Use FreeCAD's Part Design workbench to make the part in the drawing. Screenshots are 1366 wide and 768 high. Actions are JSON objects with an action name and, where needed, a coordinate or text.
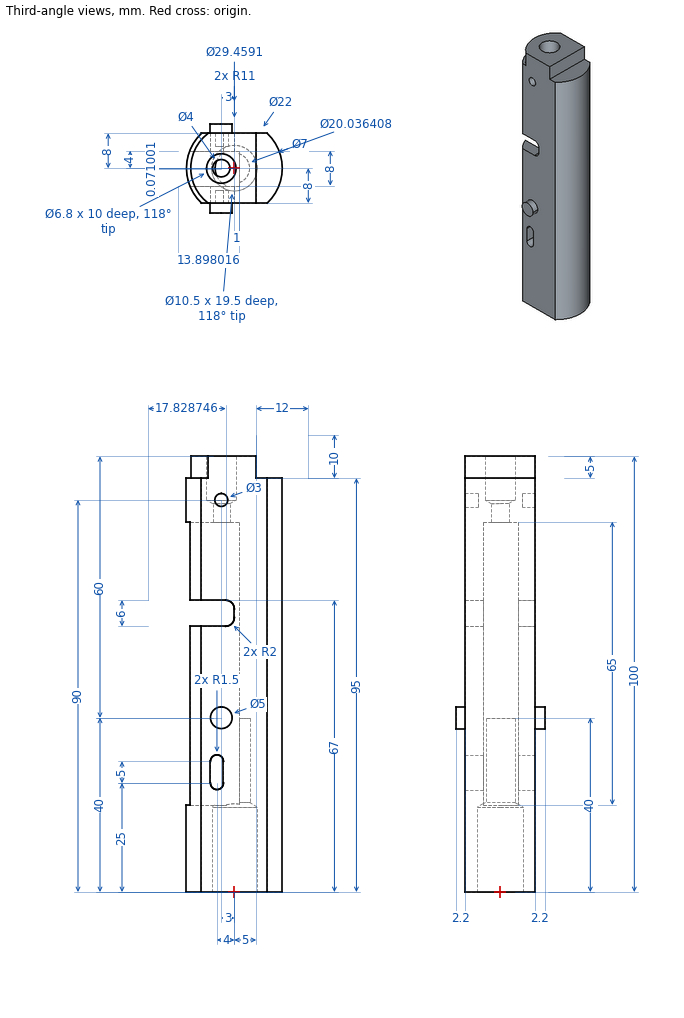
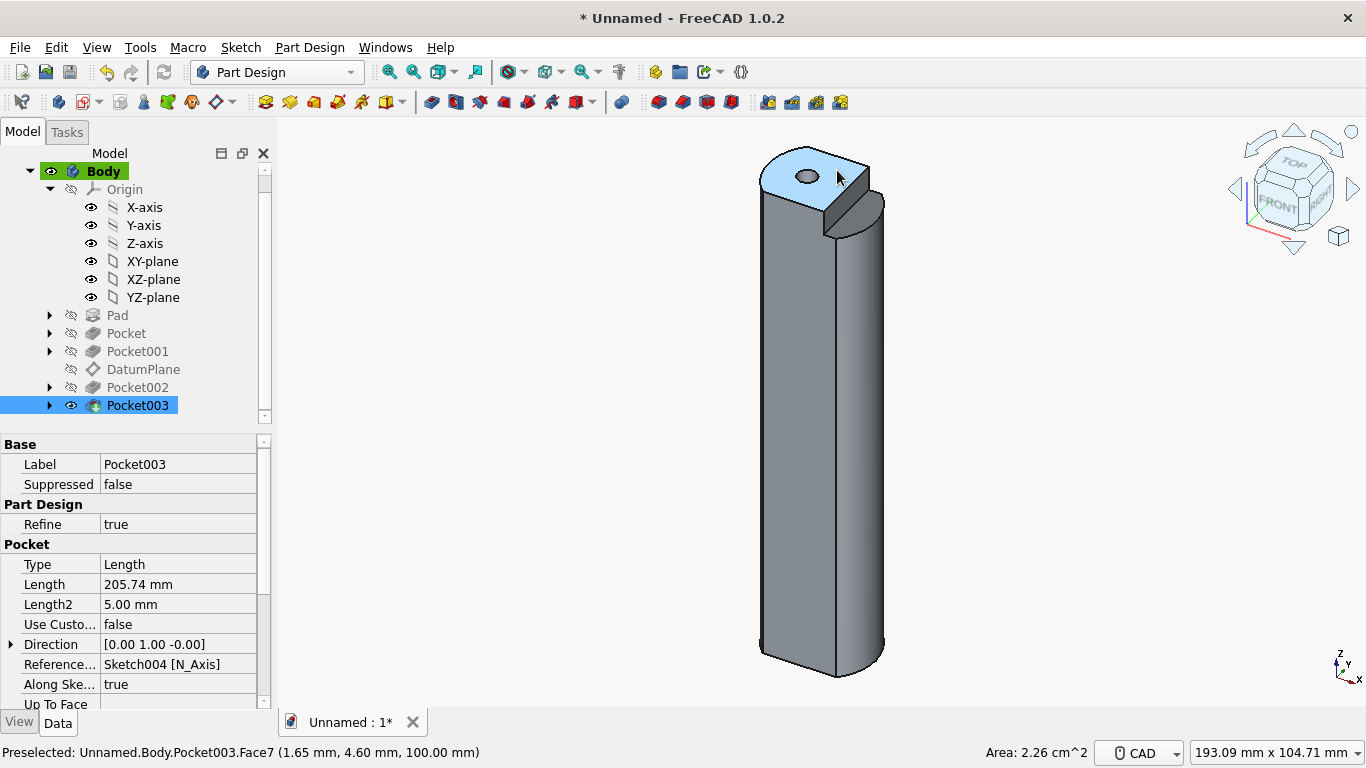
{"action": "left_click", "coordinate": [84, 102]}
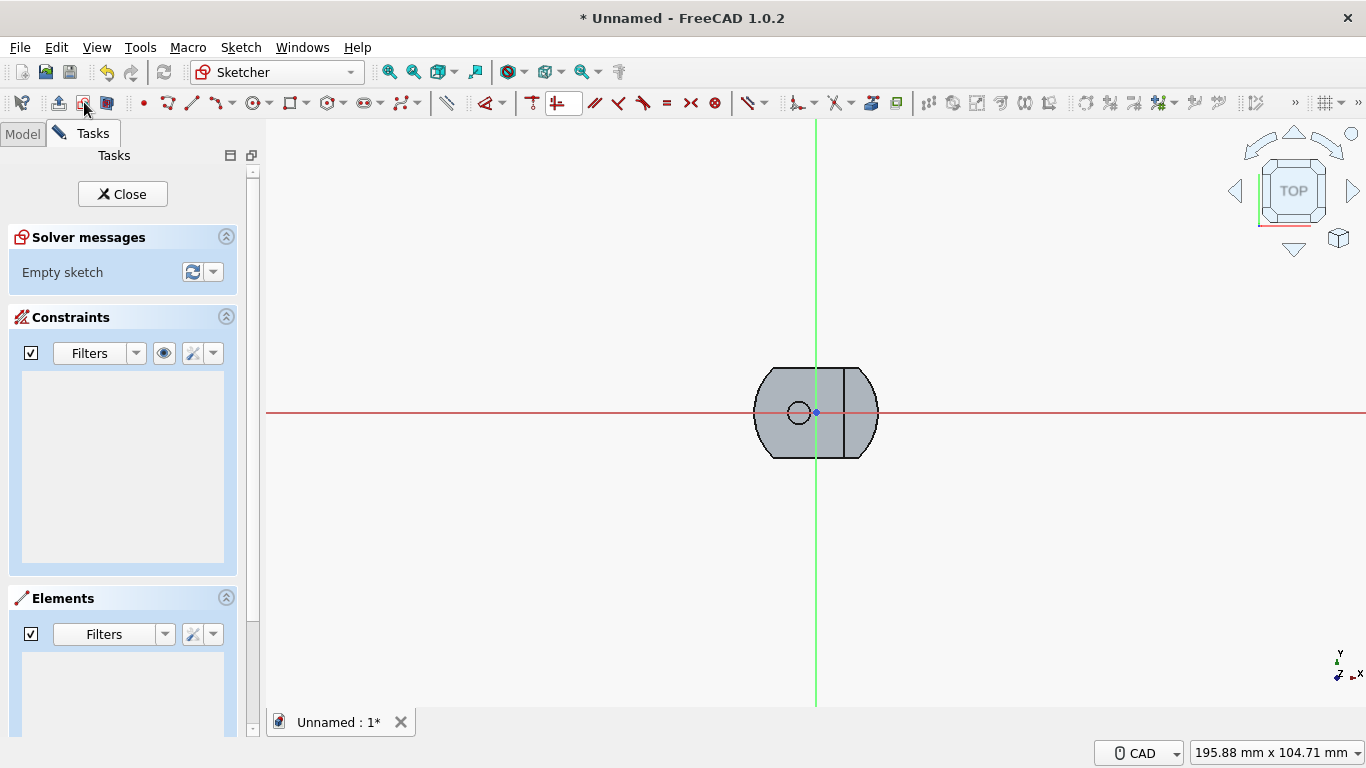
{"action": "scroll", "coordinate": [806, 413], "scroll_direction": "up", "scroll_amount": 11}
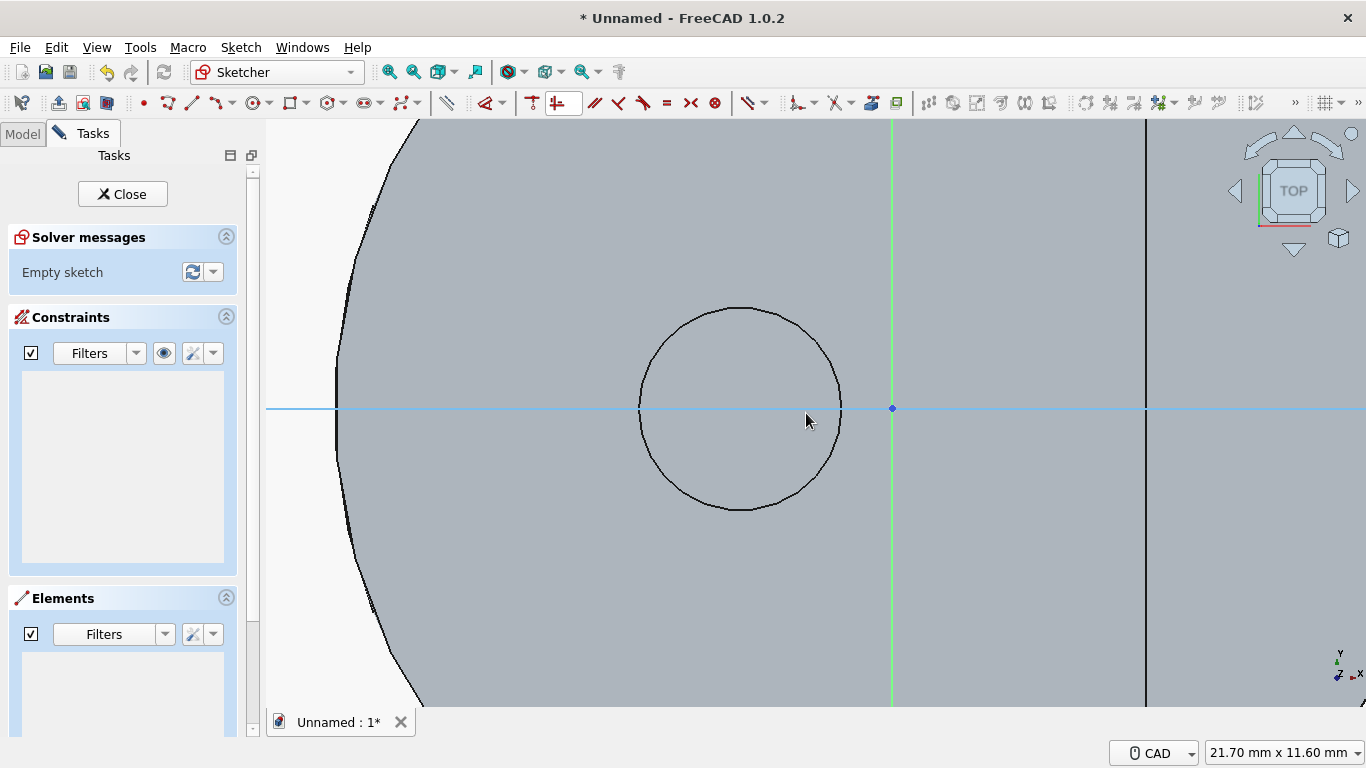
{"action": "left_click", "coordinate": [254, 104]}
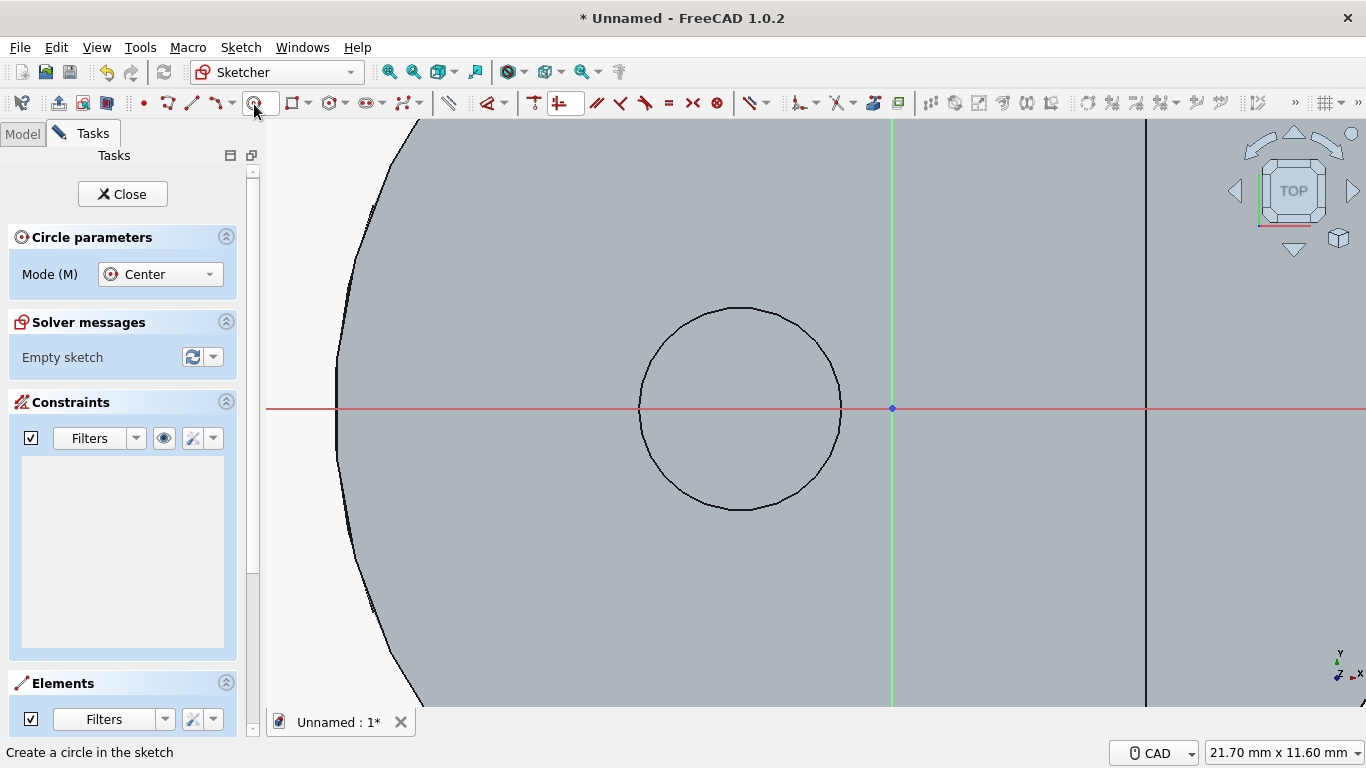
{"action": "scroll", "coordinate": [740, 413], "scroll_direction": "up", "scroll_amount": 8}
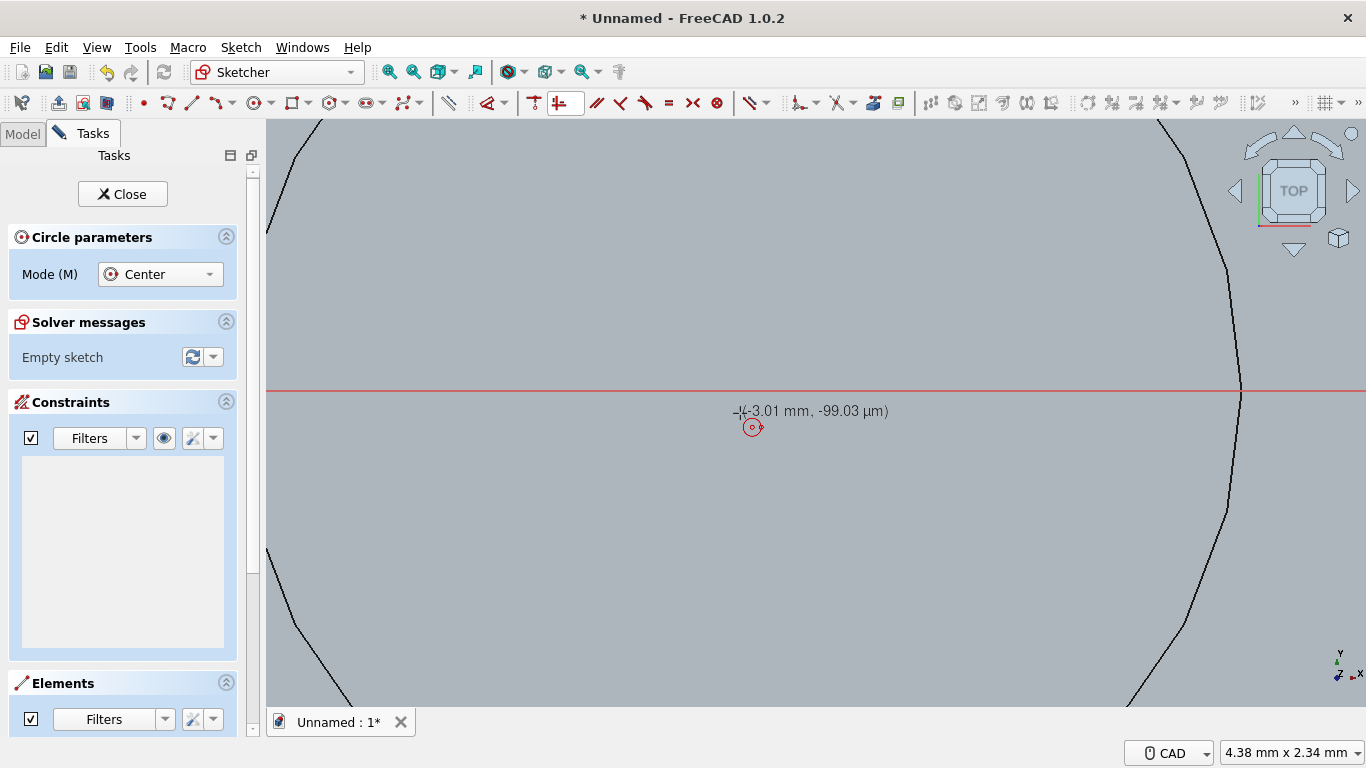
{"action": "left_click", "coordinate": [740, 409]}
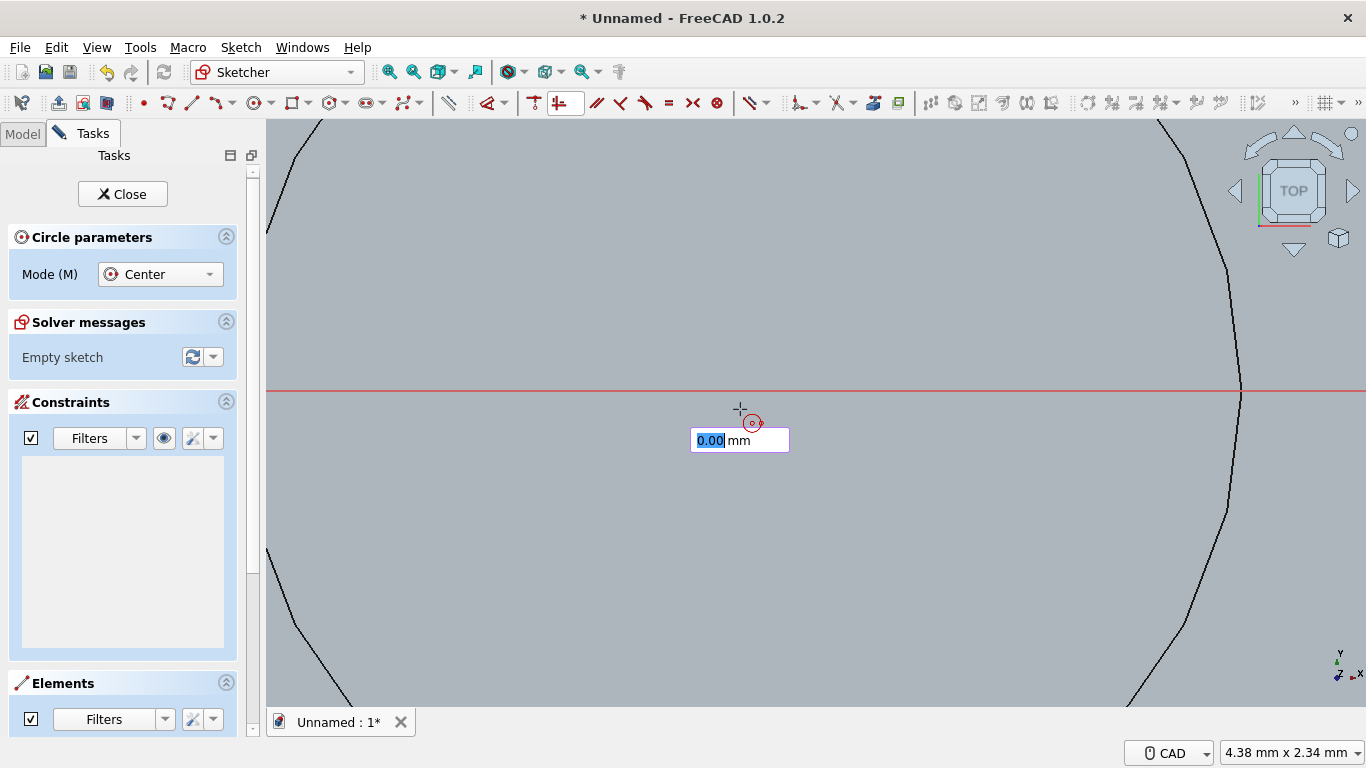
{"action": "scroll", "coordinate": [749, 414], "scroll_direction": "down", "scroll_amount": 8}
{"action": "mouse_move", "coordinate": [869, 292]}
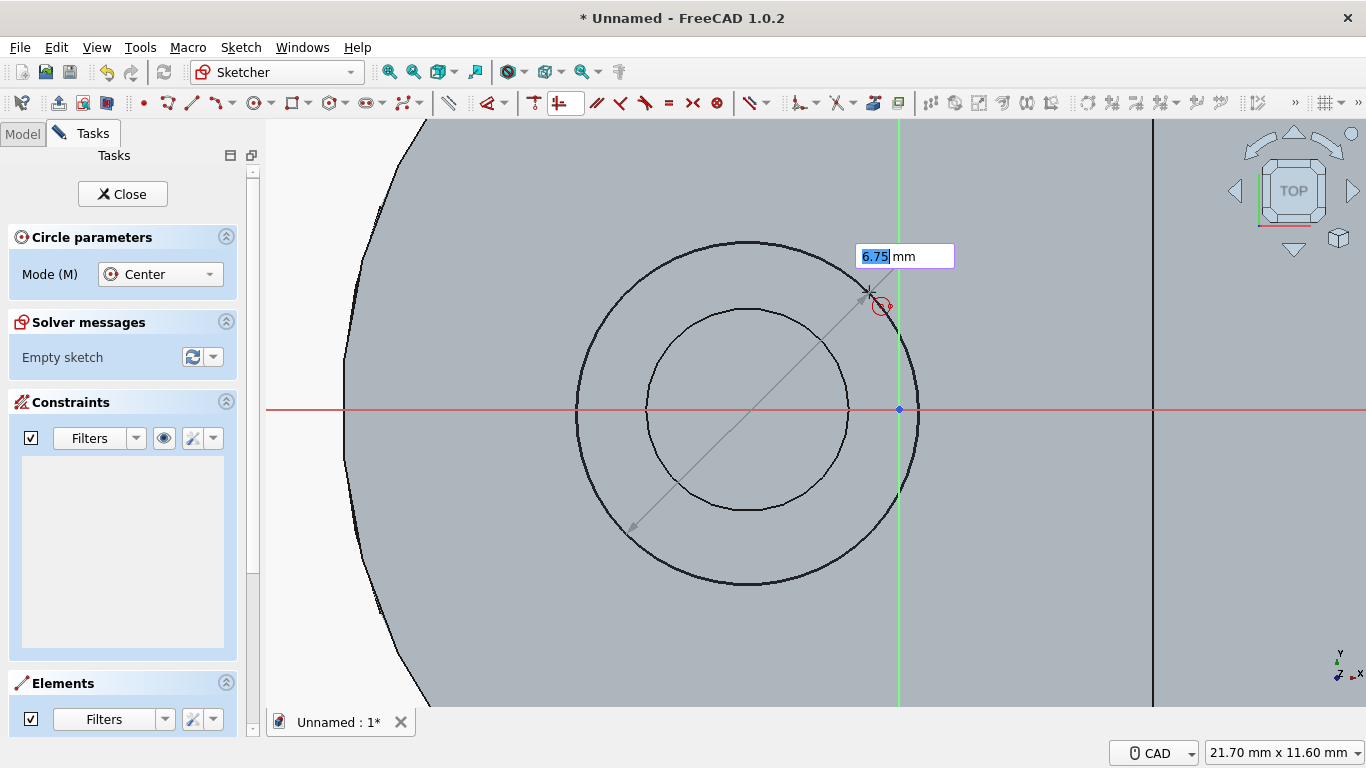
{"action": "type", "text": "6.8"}
{"action": "key", "text": "Return"}
{"action": "key", "text": "Escape"}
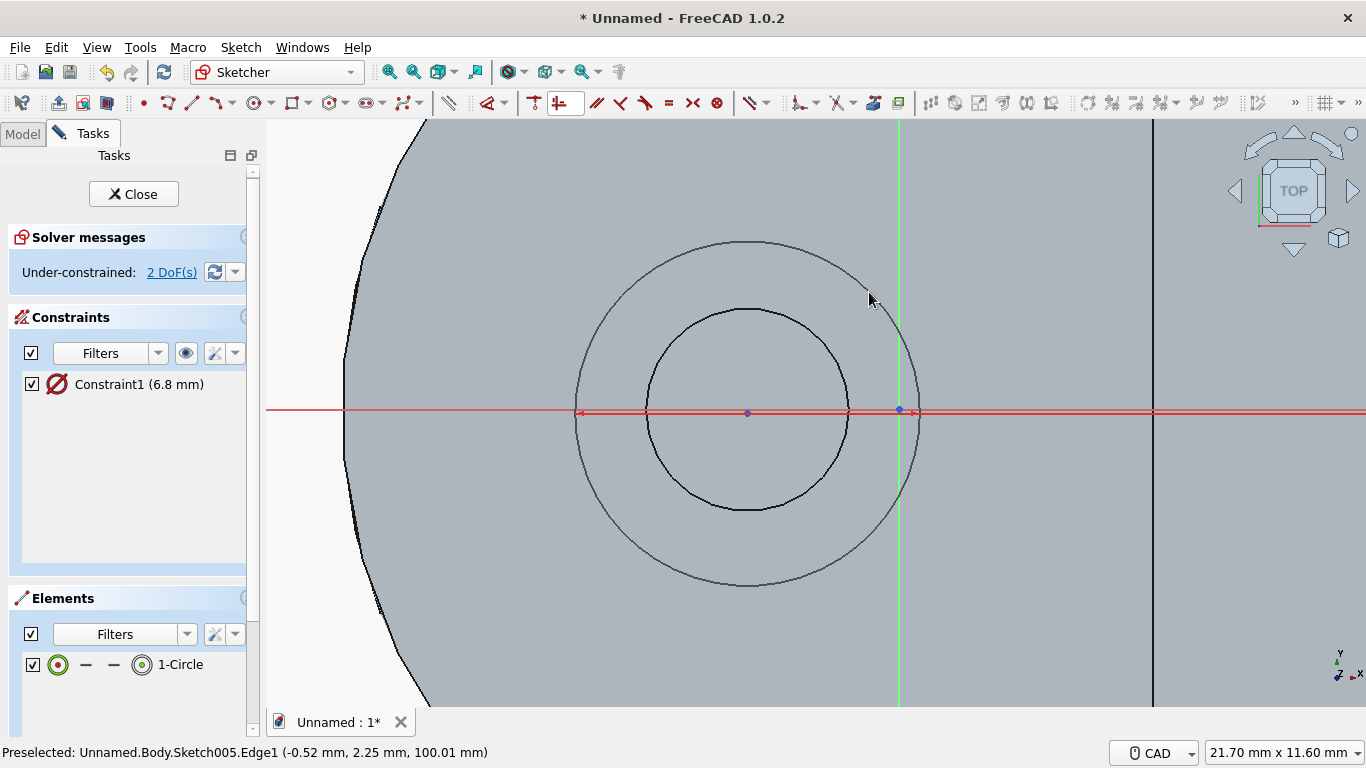
{"action": "key", "text": "d"}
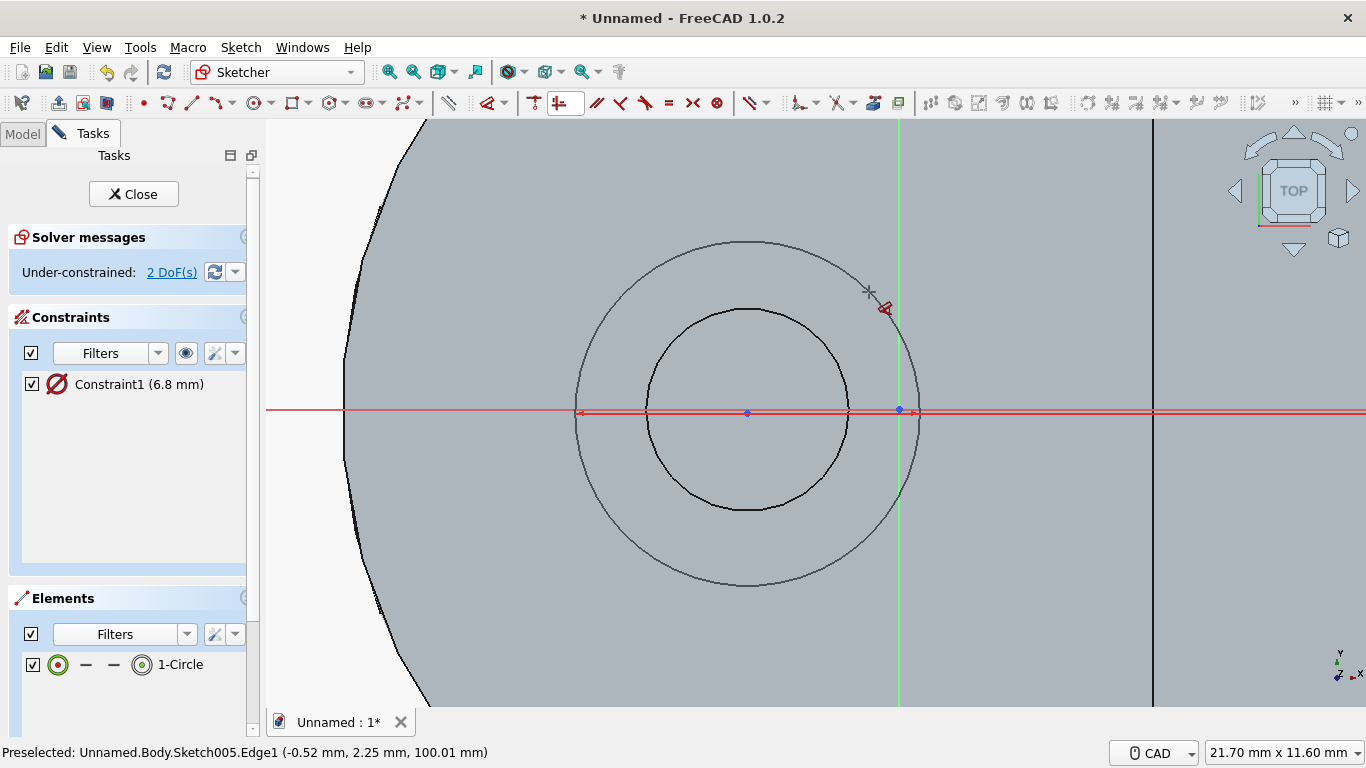
{"action": "left_click", "coordinate": [748, 414]}
{"action": "left_click", "coordinate": [824, 376]}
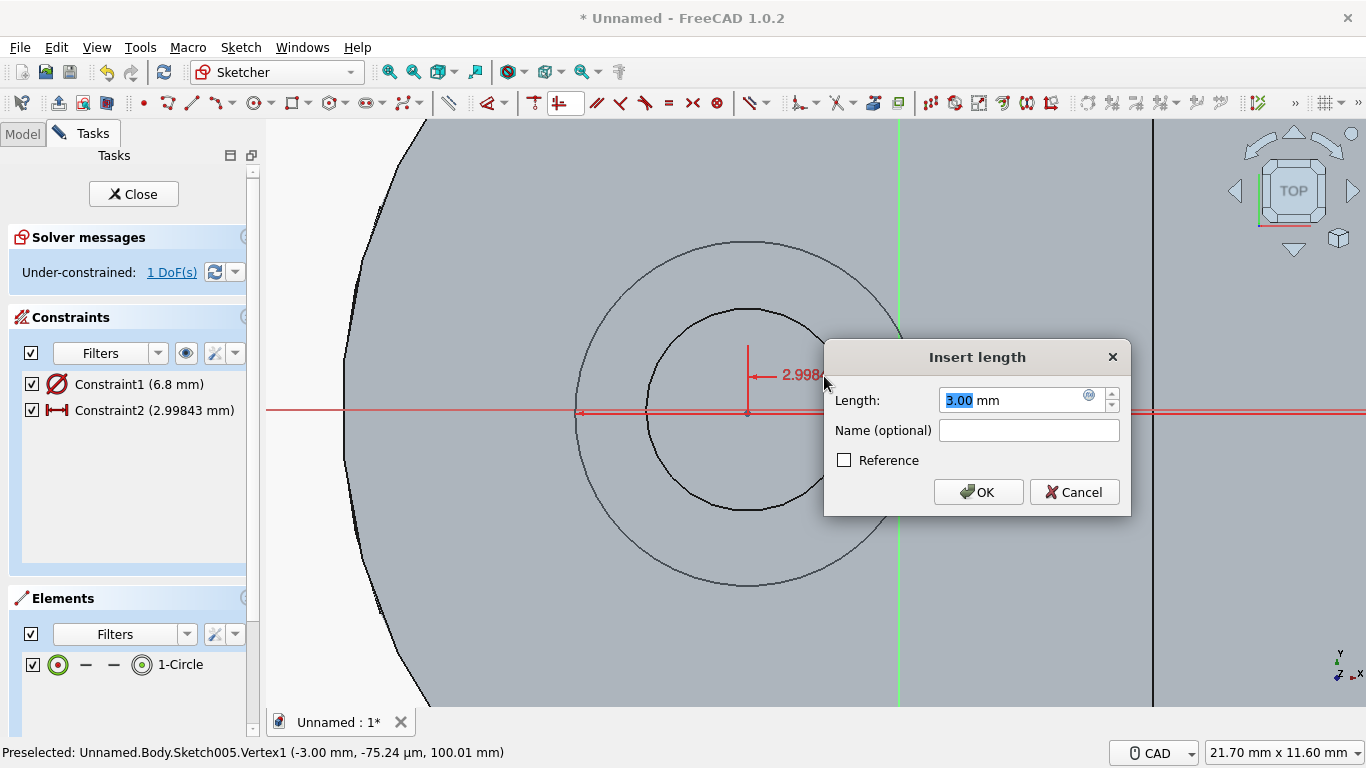
{"action": "type", "text": "3"}
{"action": "key", "text": "Return"}